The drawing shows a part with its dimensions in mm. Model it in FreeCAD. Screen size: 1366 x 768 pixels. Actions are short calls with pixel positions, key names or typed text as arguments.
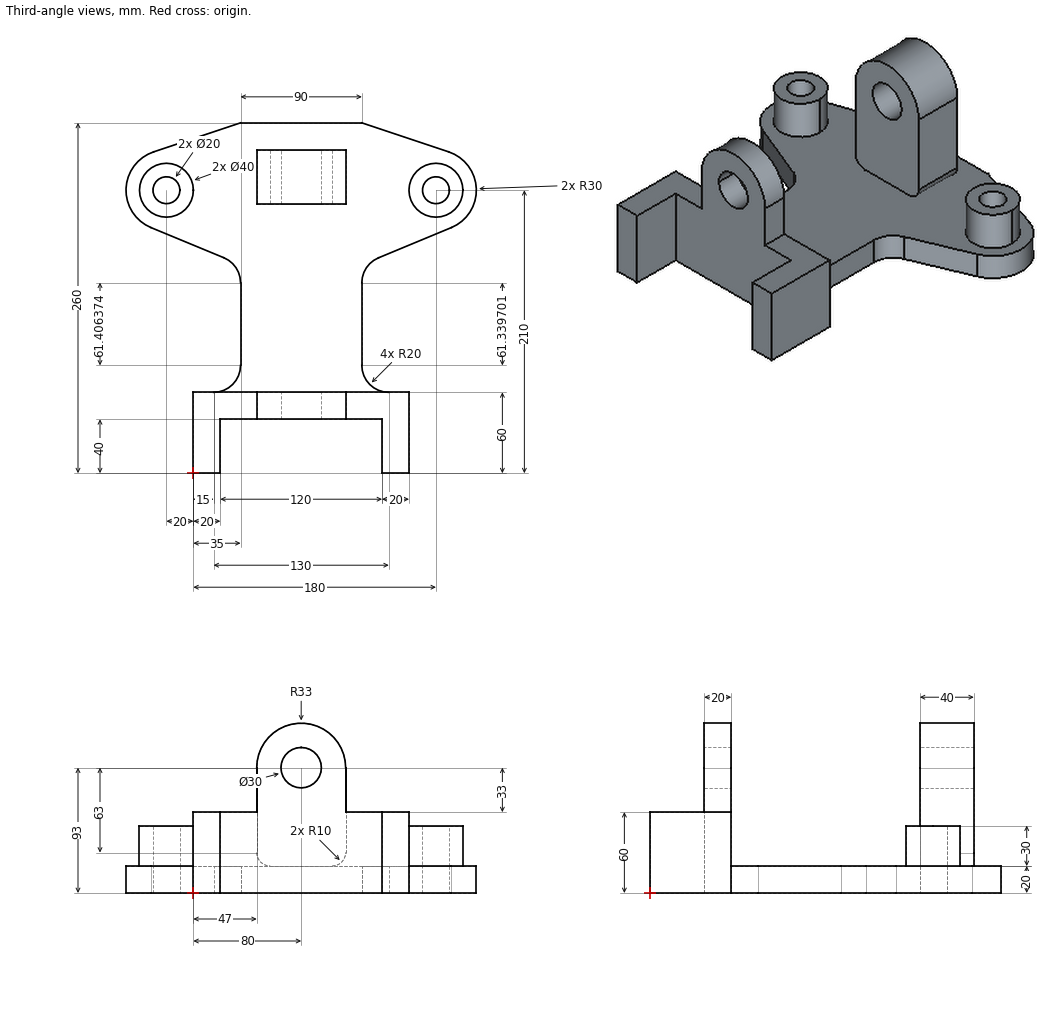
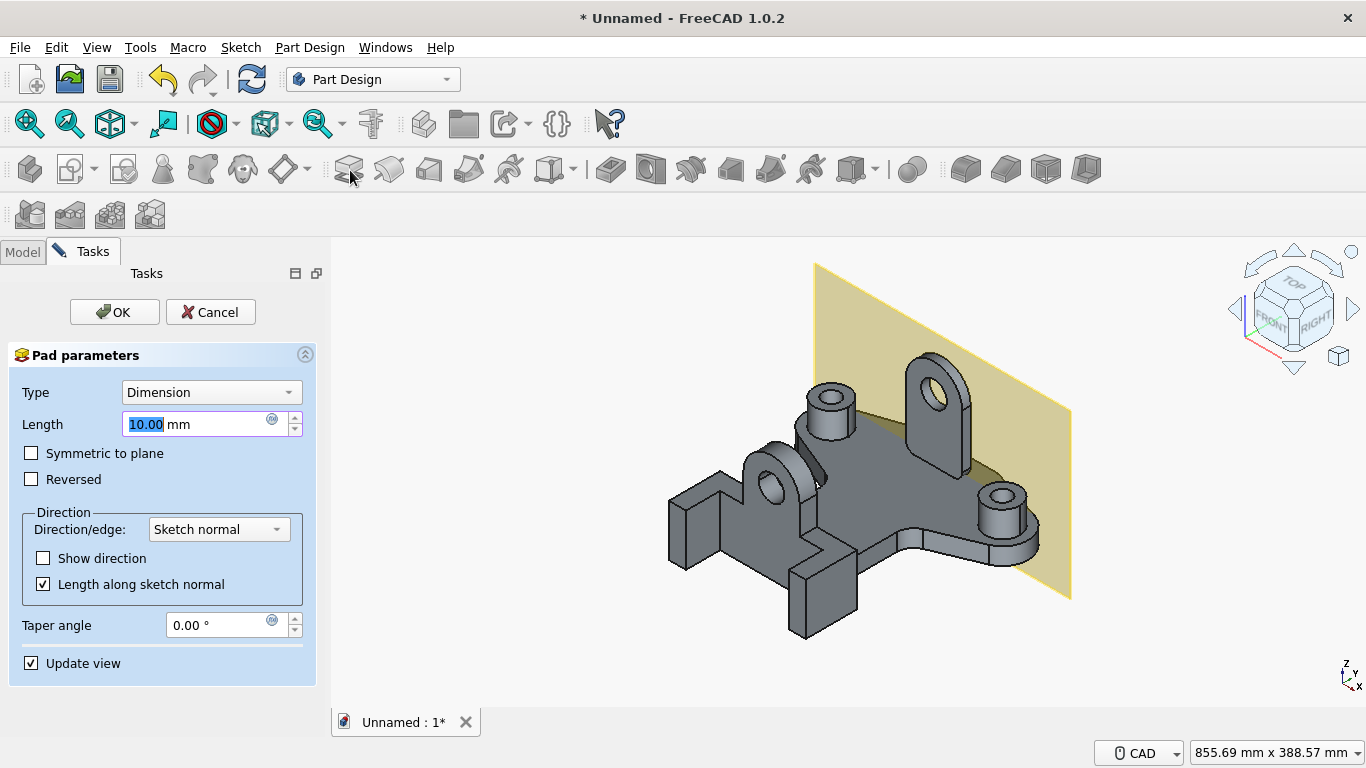
text(40)
key(Tab)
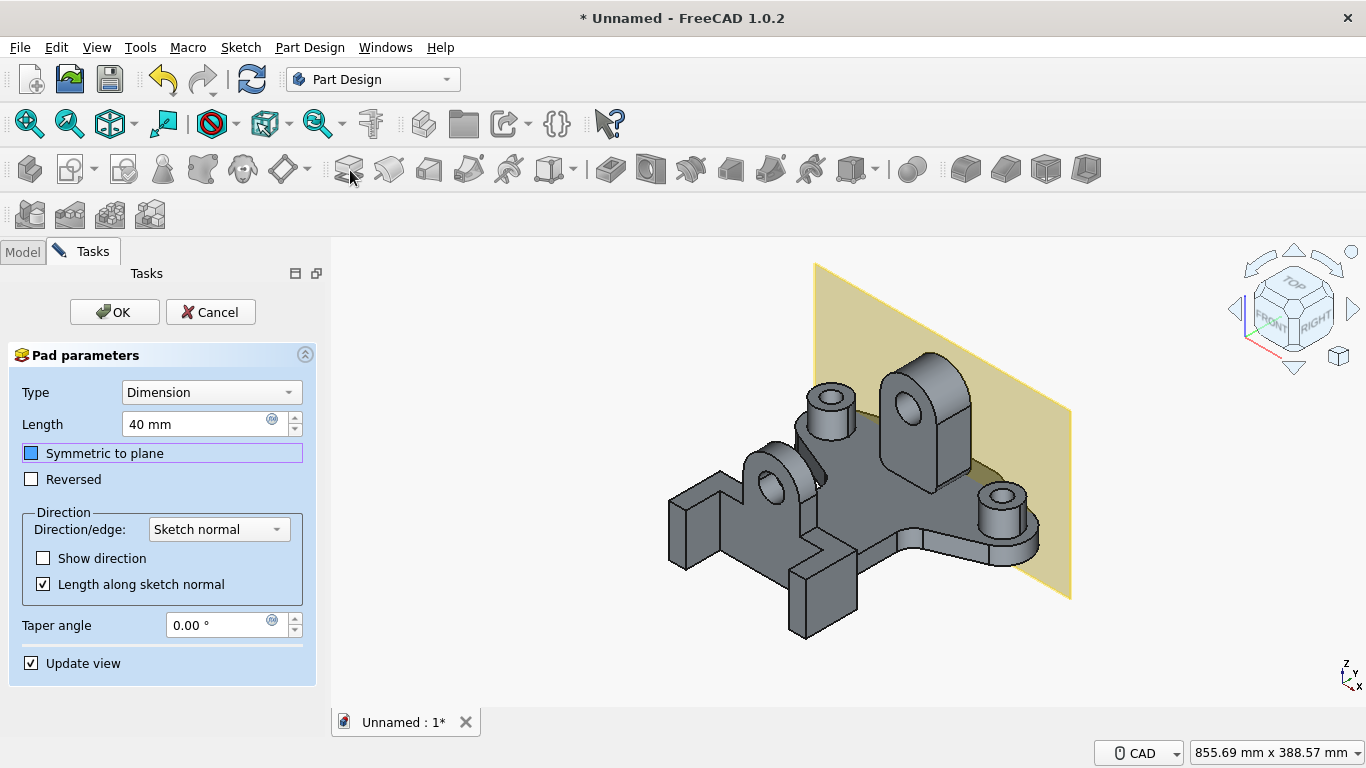
click(115, 312)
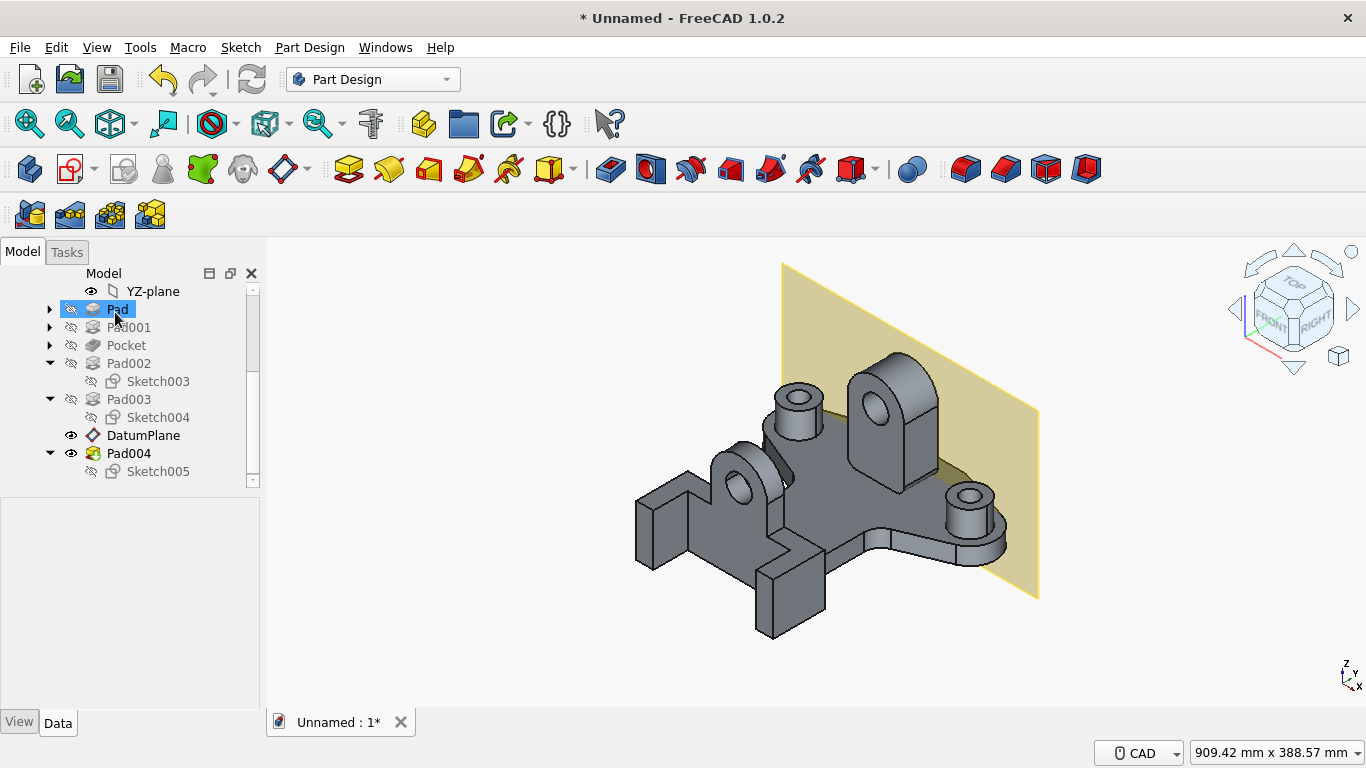
click(116, 435)
key(space)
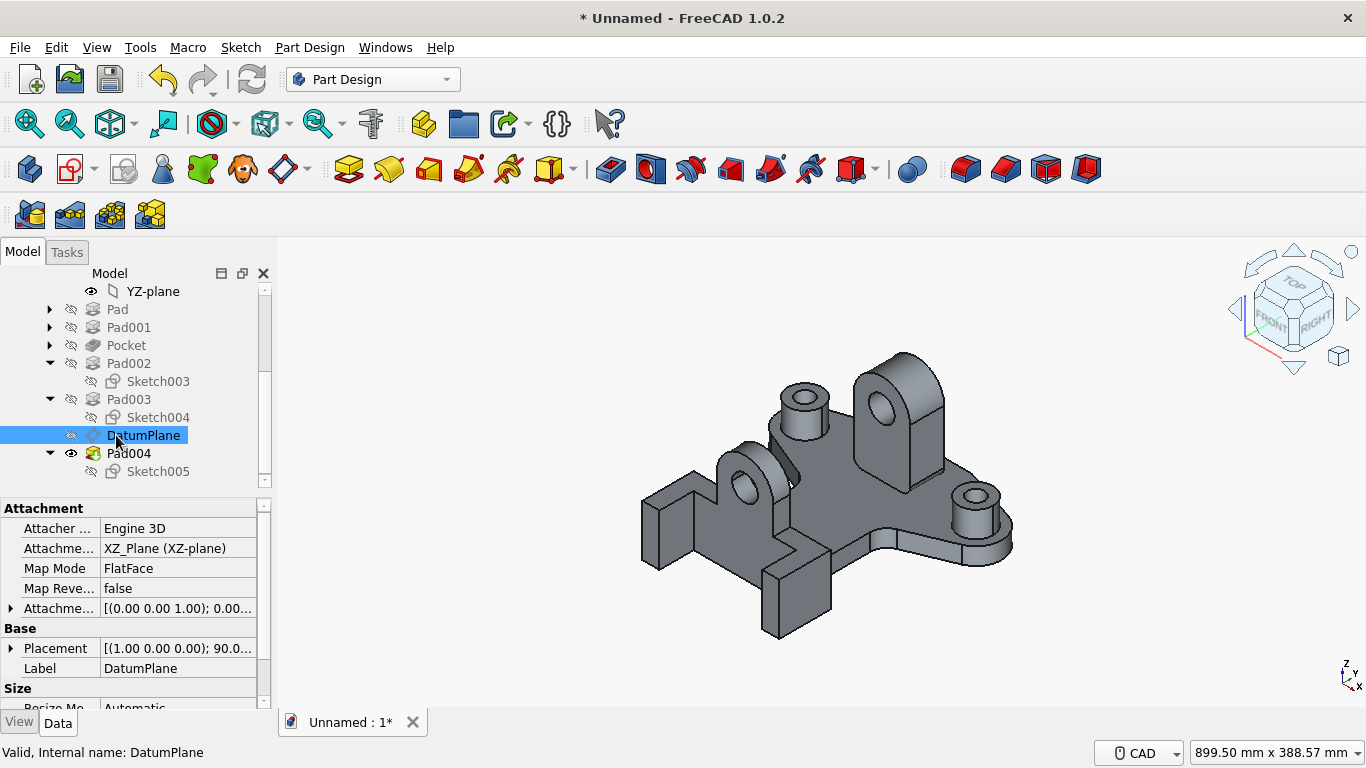
scroll(160, 377, down, 3)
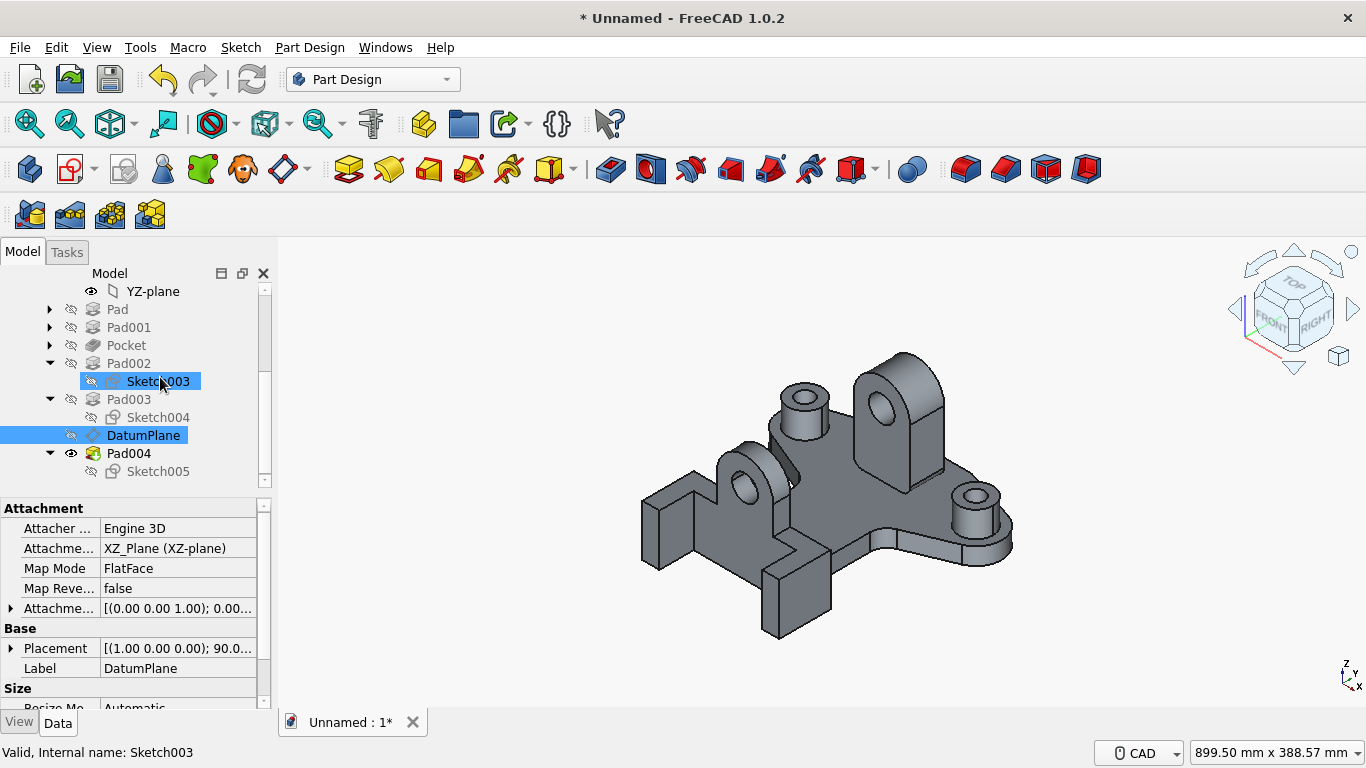
scroll(160, 377, up, 15)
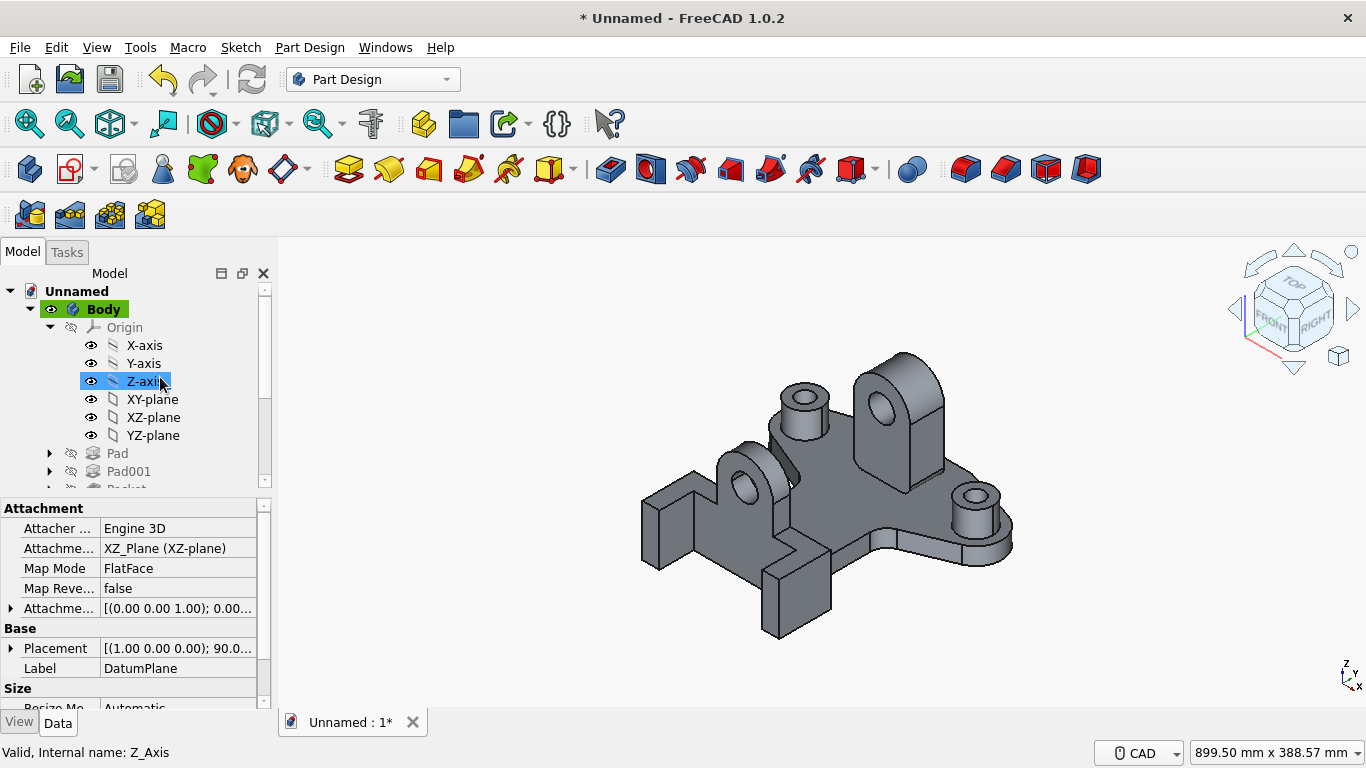
click(136, 399)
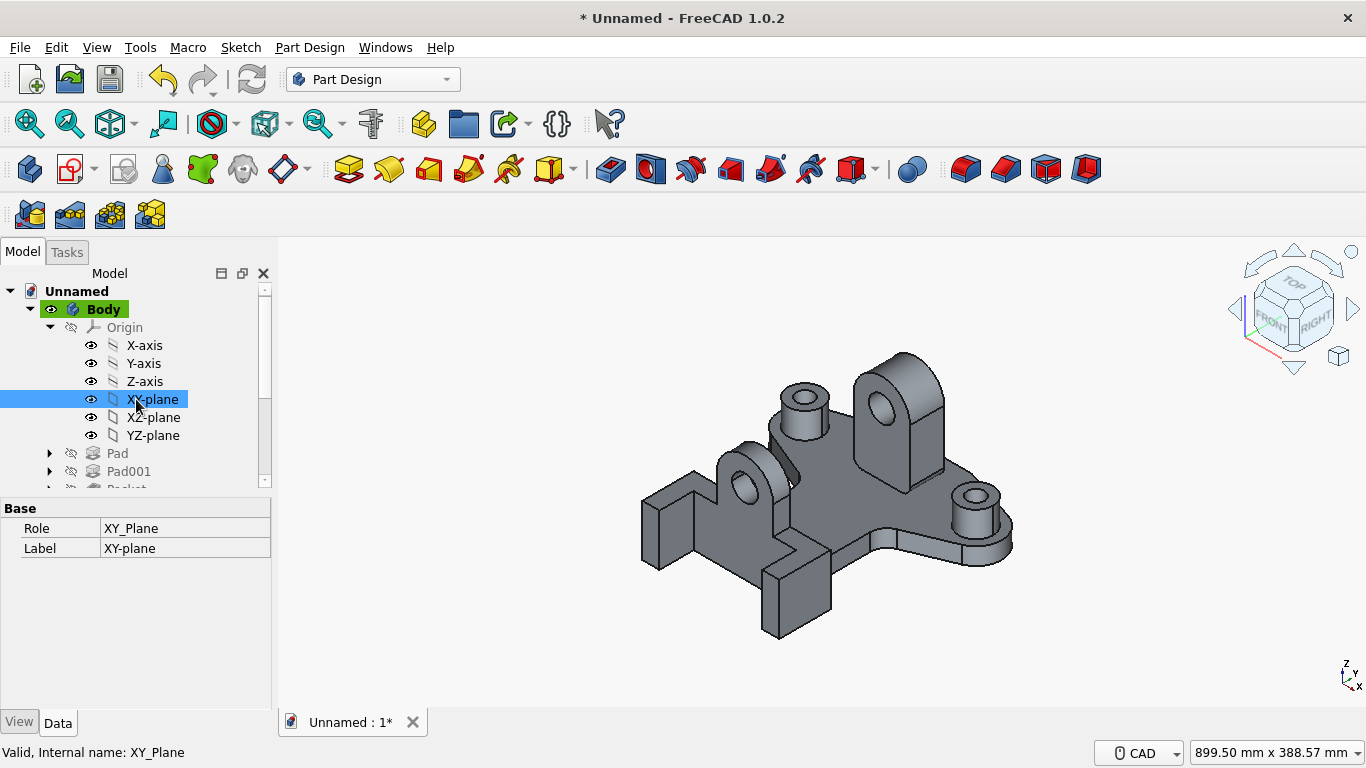
click(284, 170)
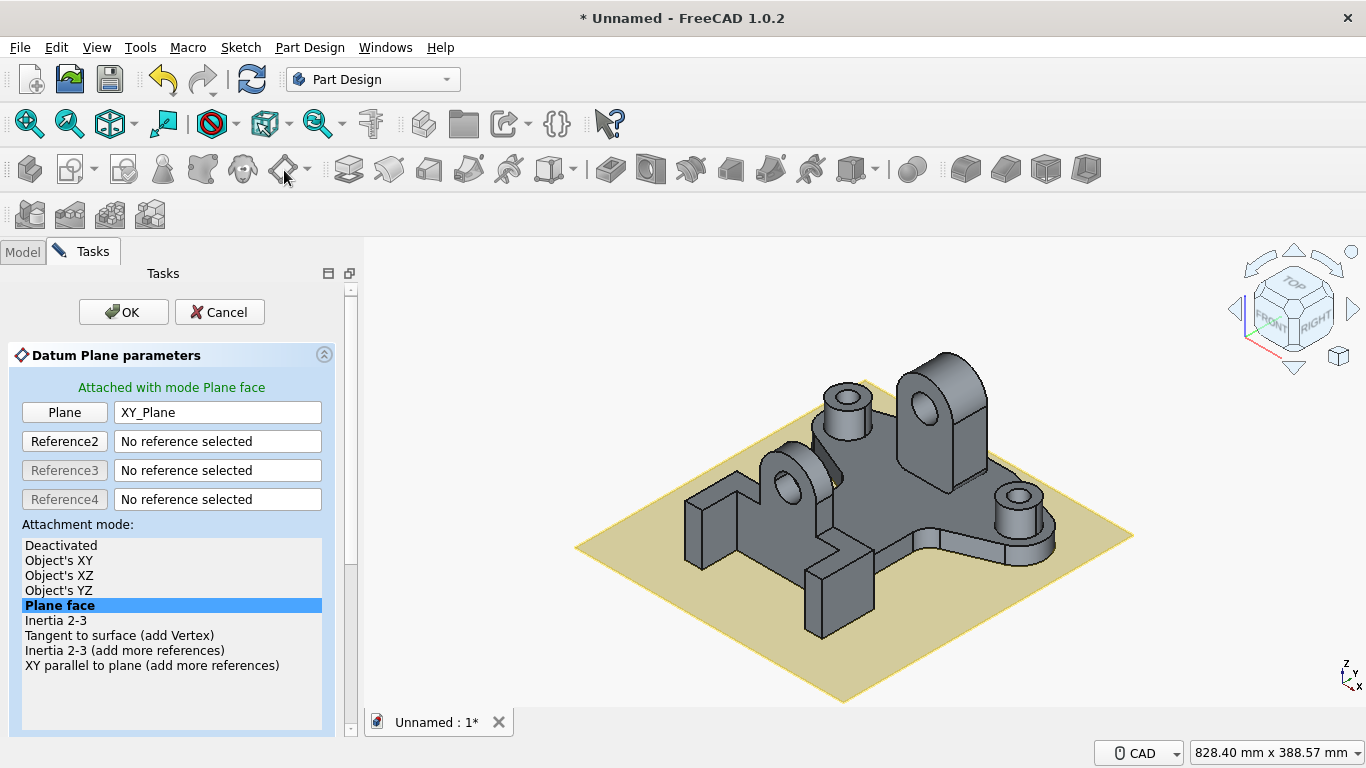
scroll(351, 510, down, 3)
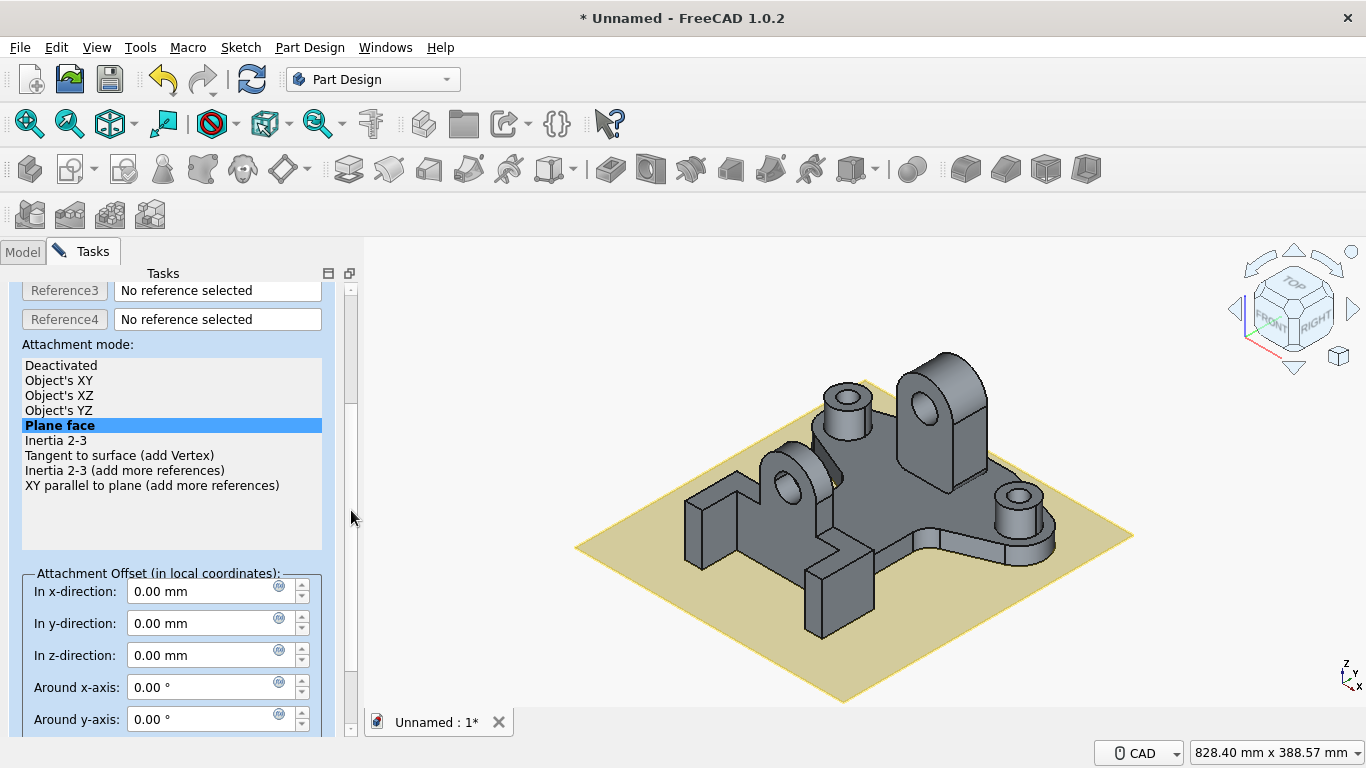
triple_click(210, 655)